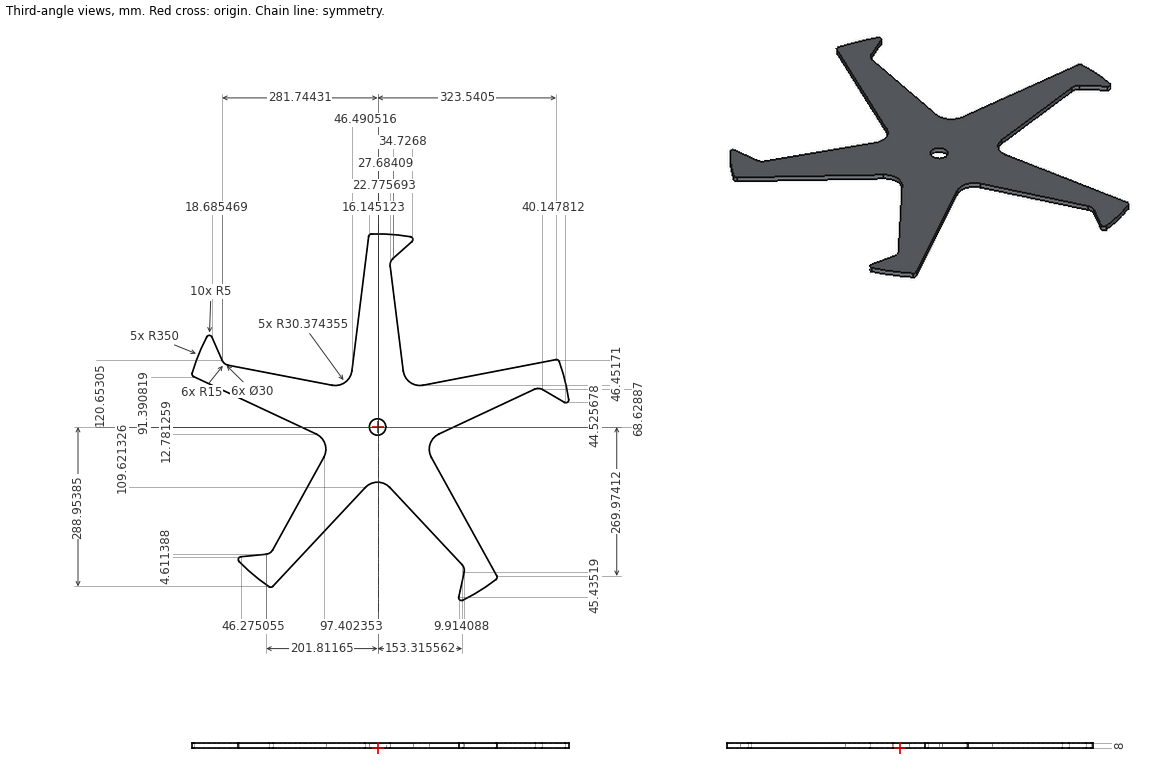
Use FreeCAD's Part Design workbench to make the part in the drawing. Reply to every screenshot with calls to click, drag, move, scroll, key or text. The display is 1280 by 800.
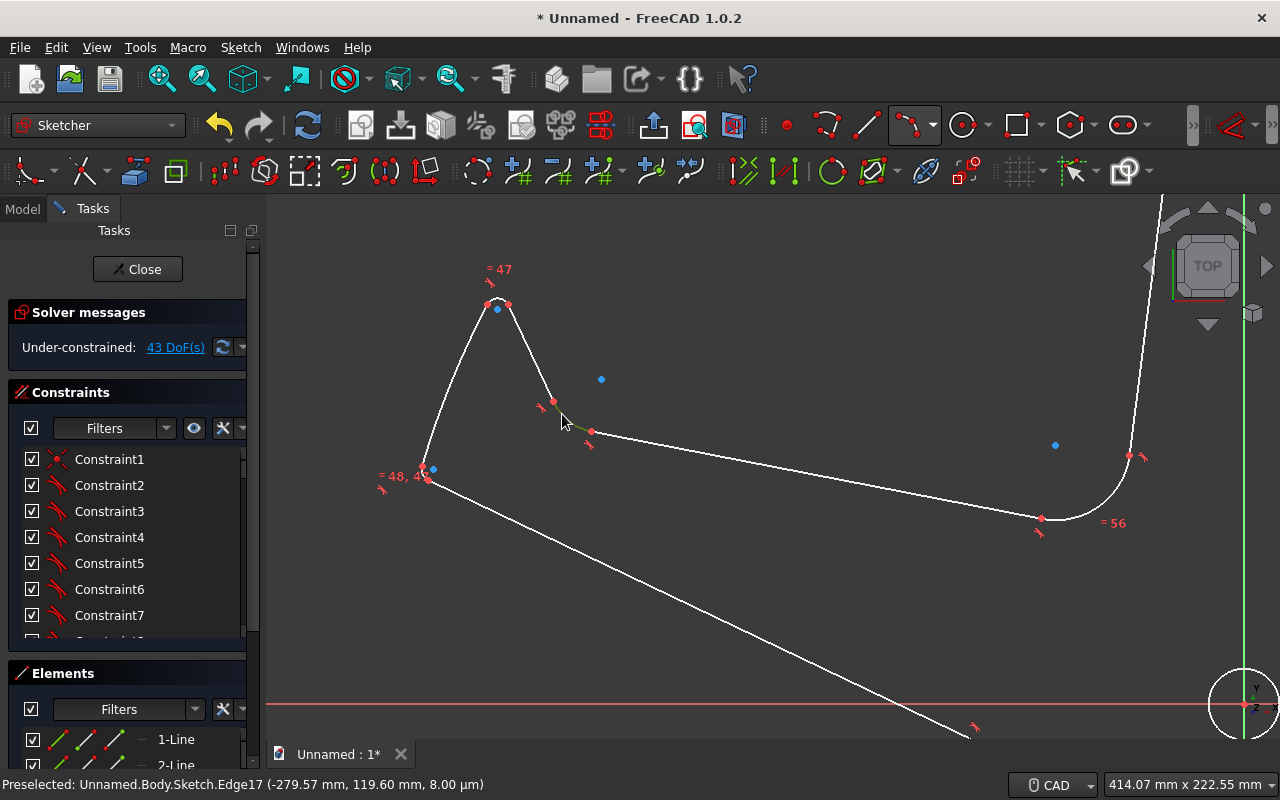
scroll(565, 417, down, 8)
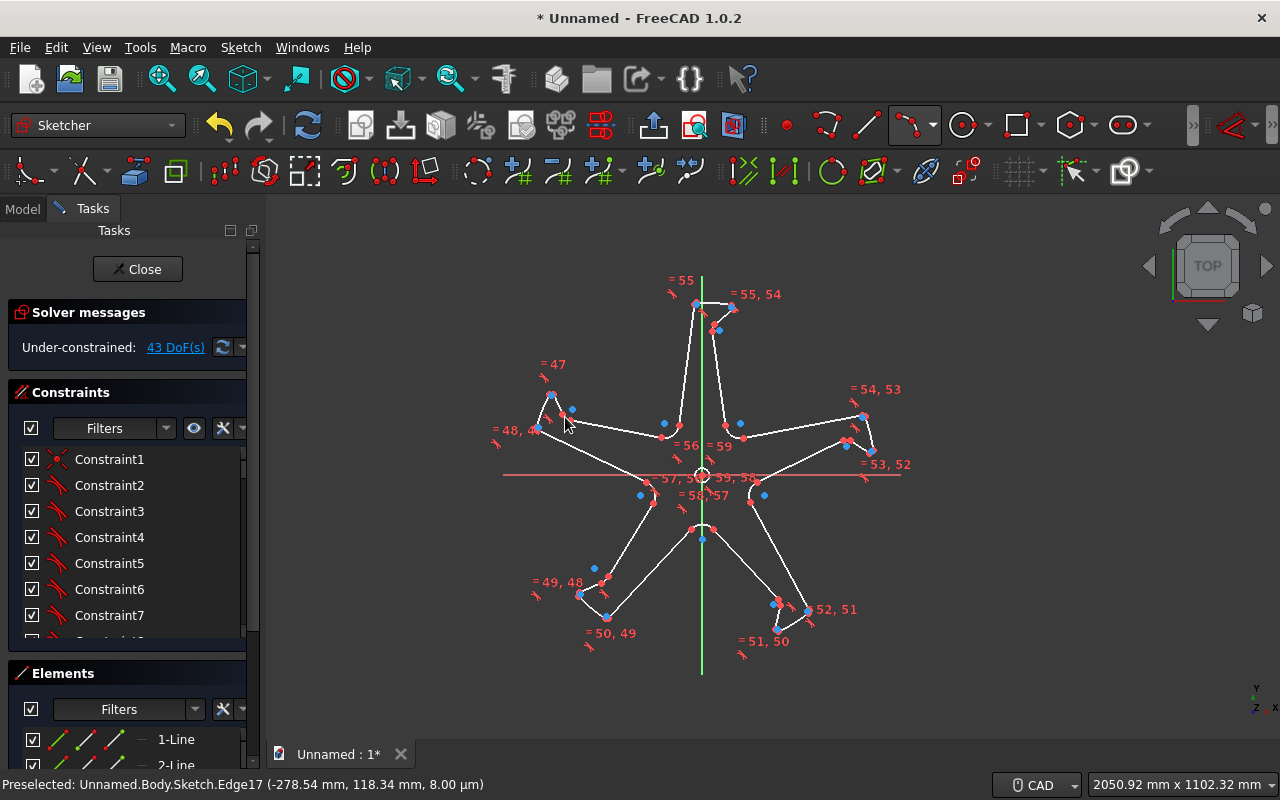
scroll(604, 582, up, 8)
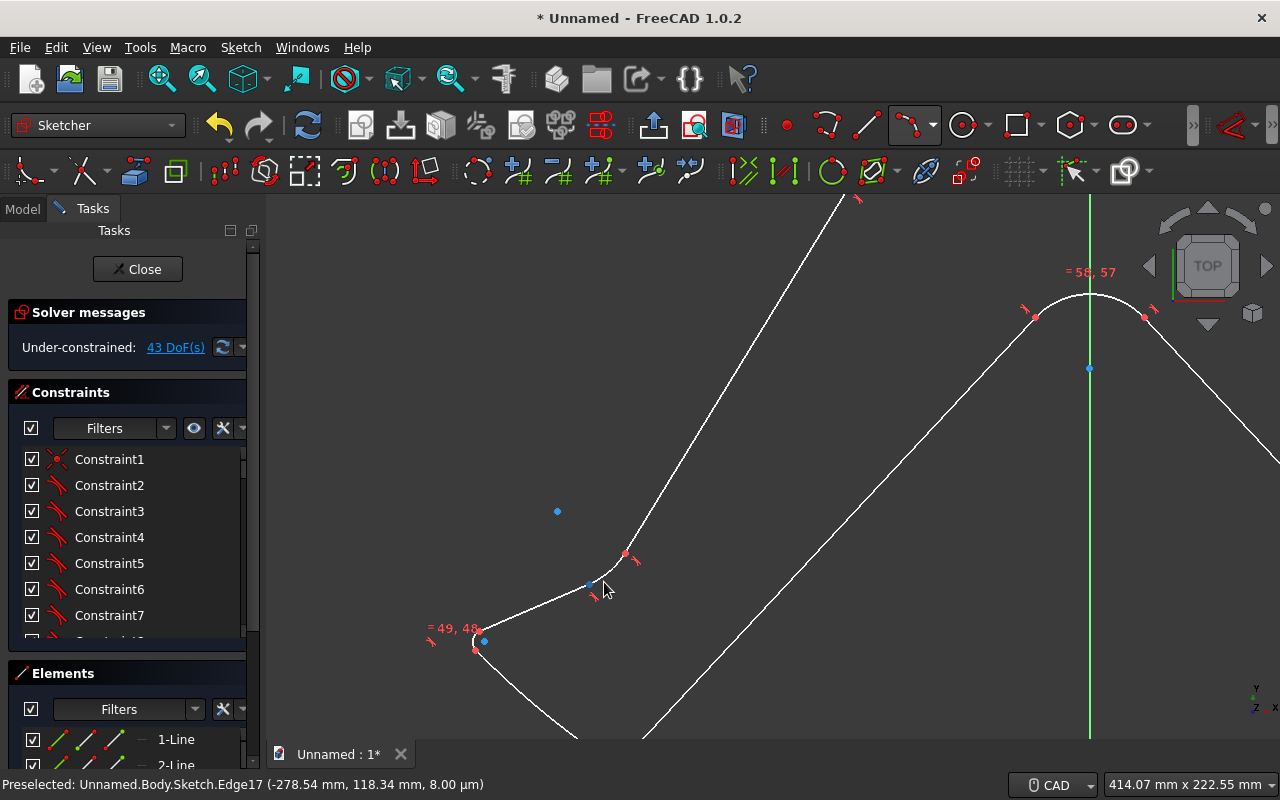
click(602, 577)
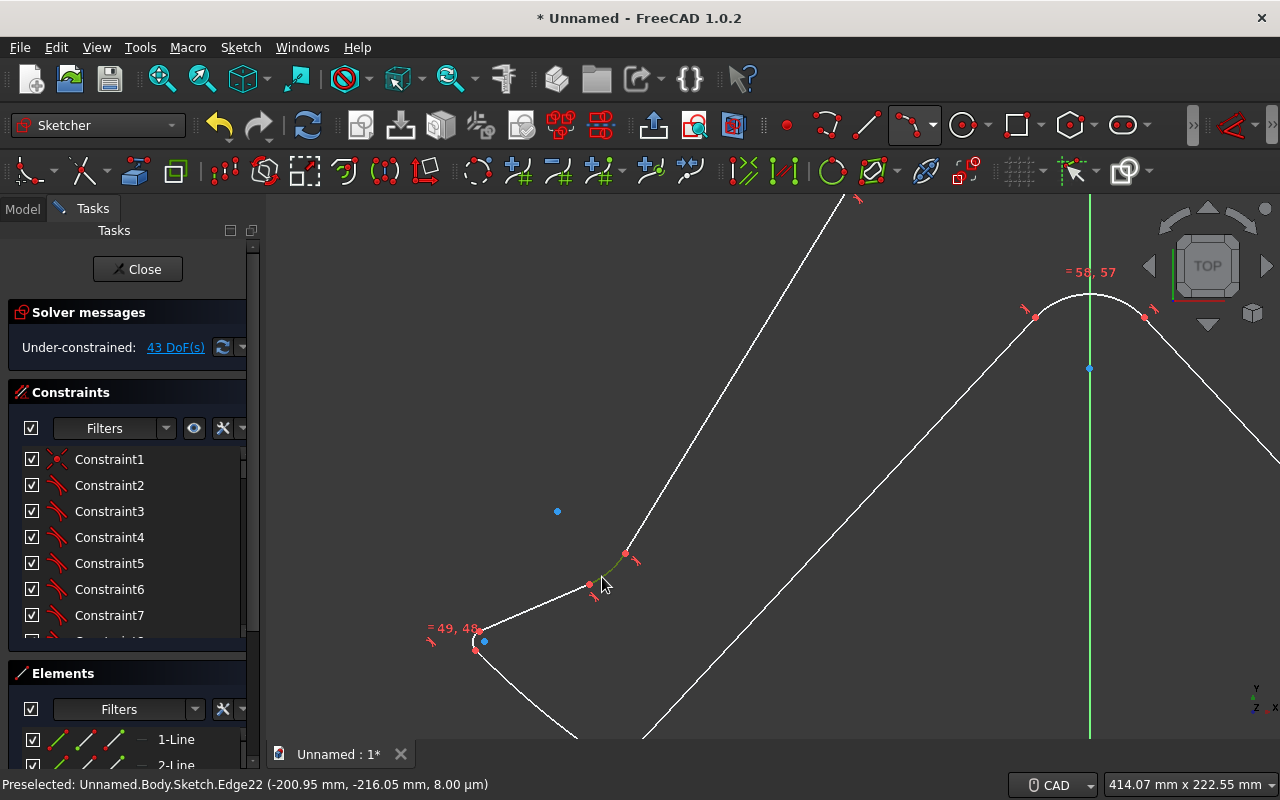
scroll(604, 583, down, 8)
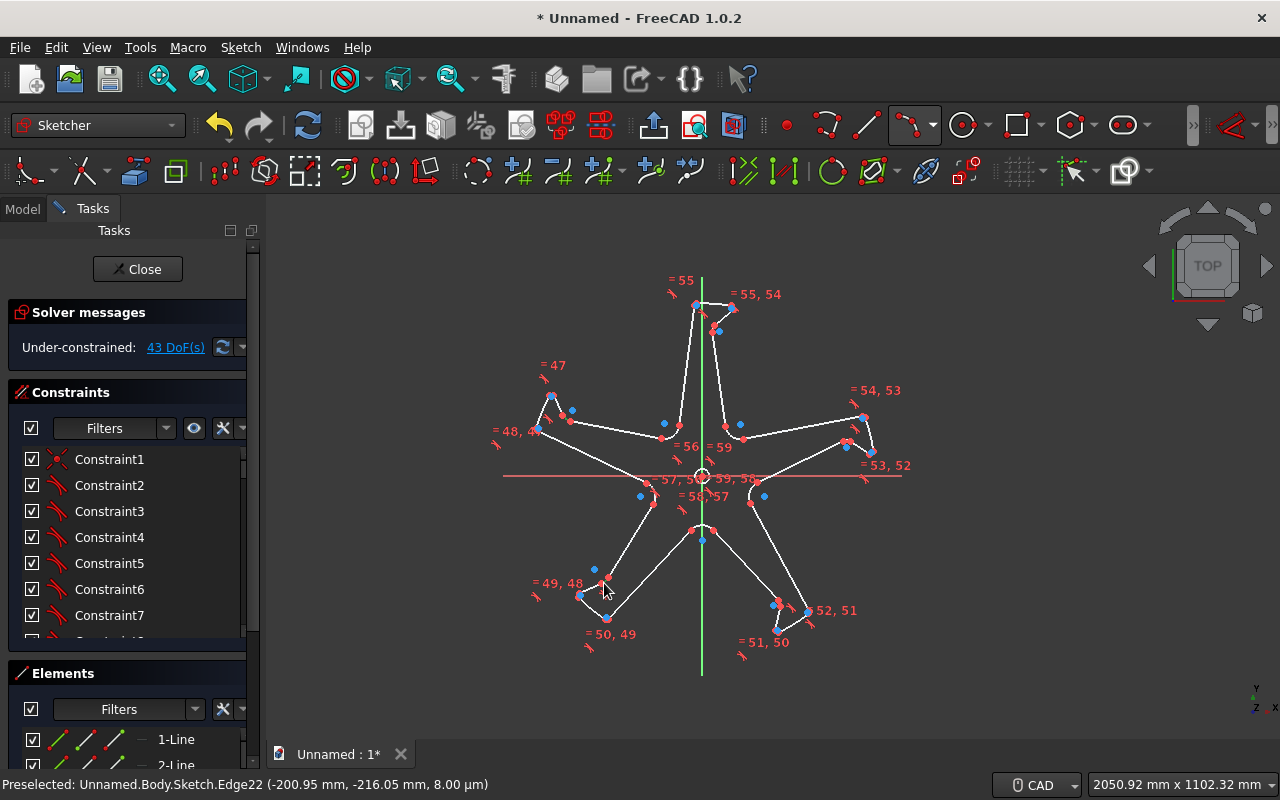
scroll(781, 605, up, 10)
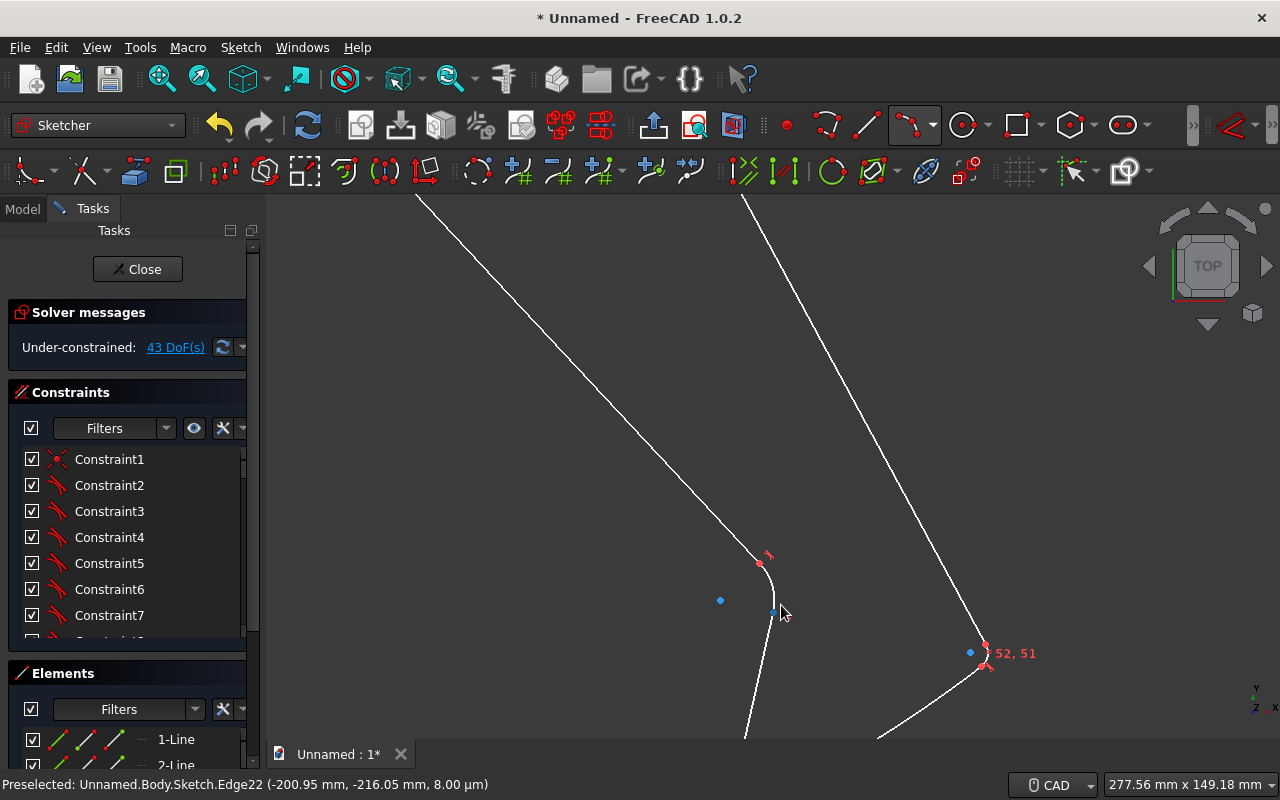
click(774, 597)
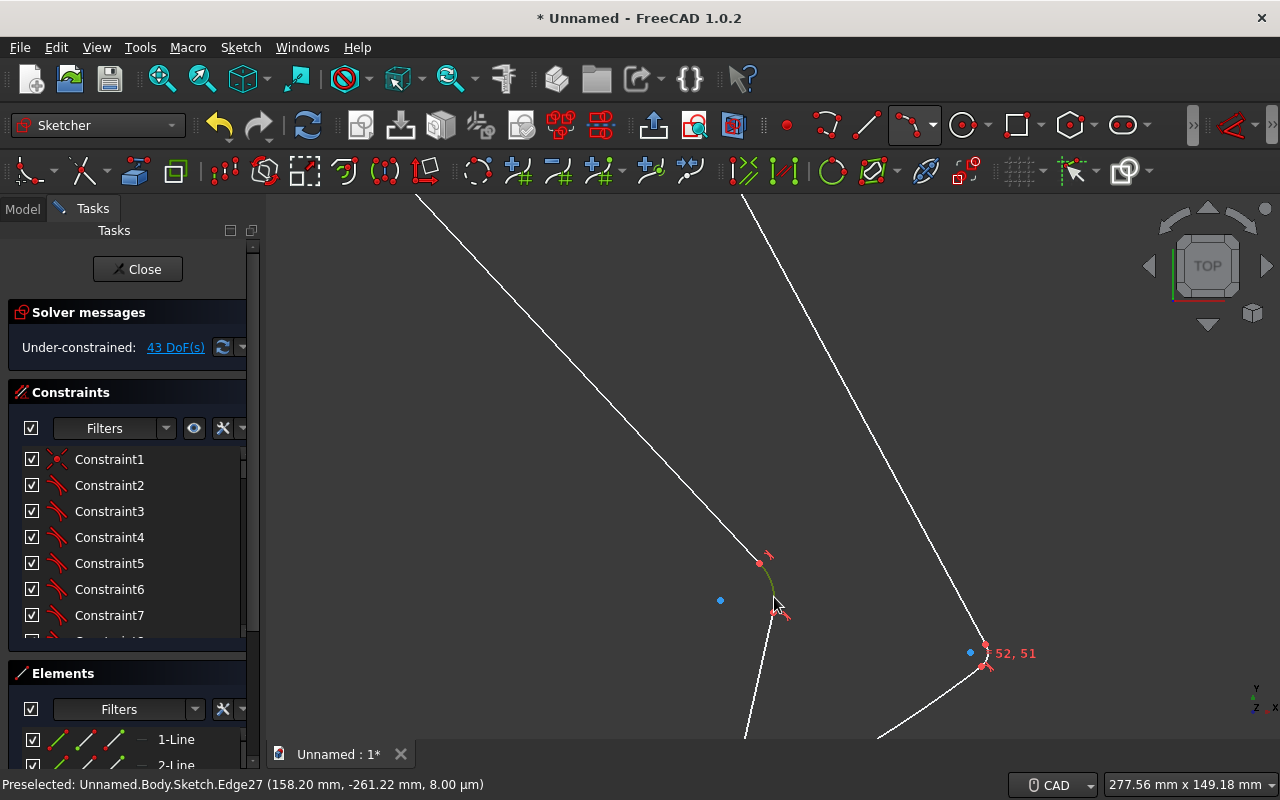
scroll(781, 605, down, 10)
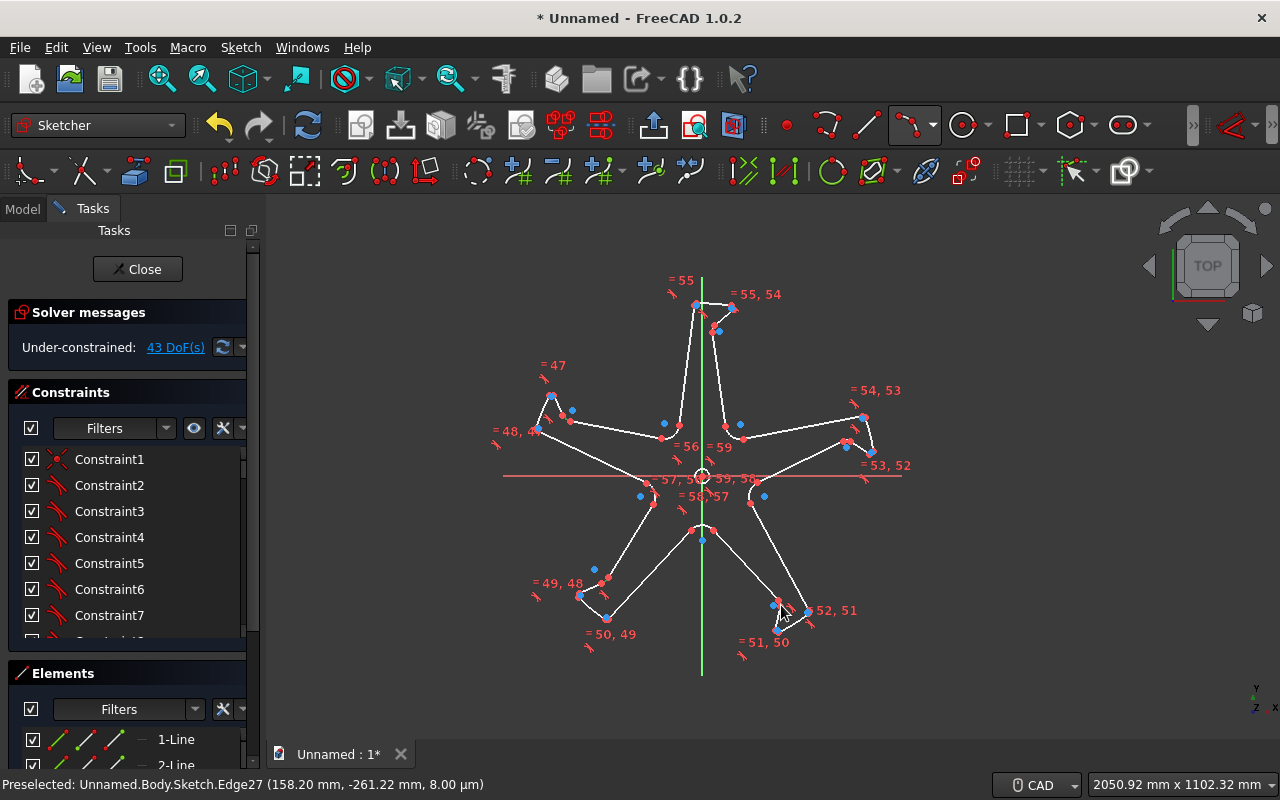
scroll(848, 441, up, 10)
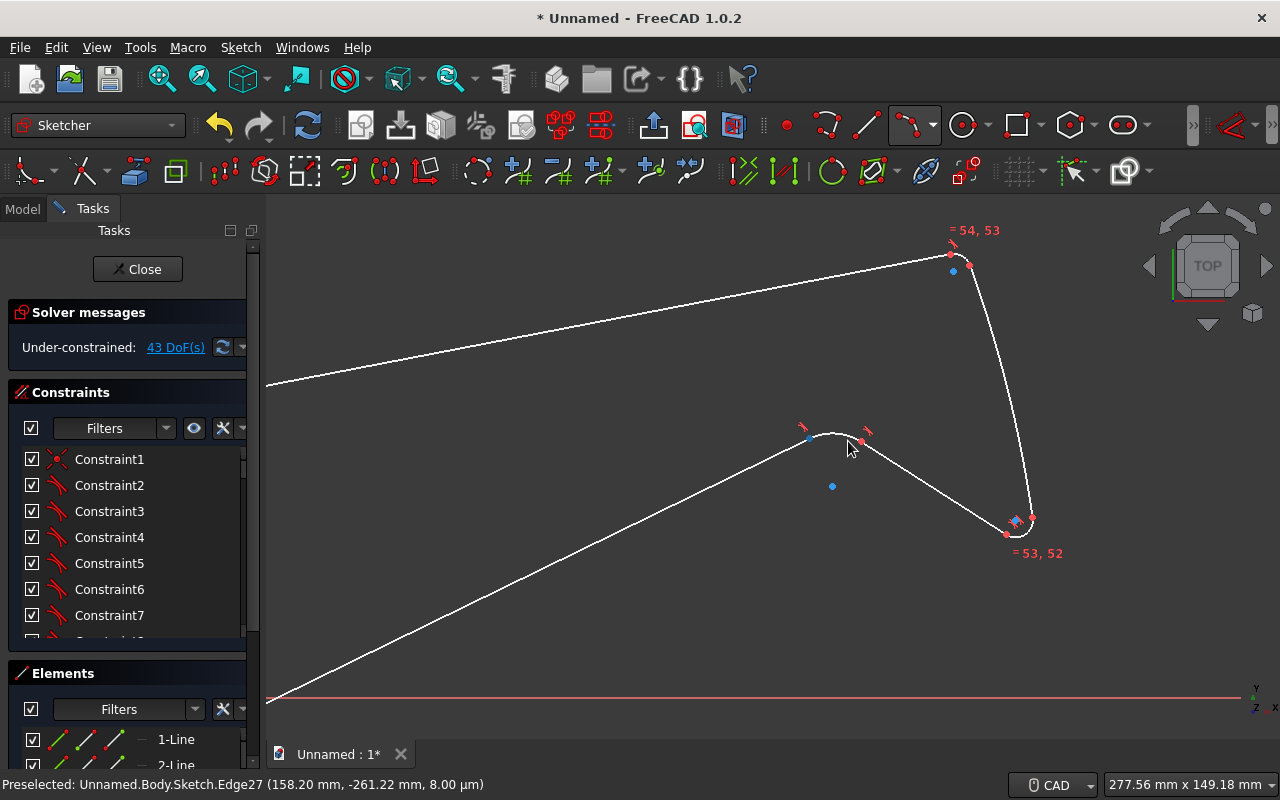
click(846, 435)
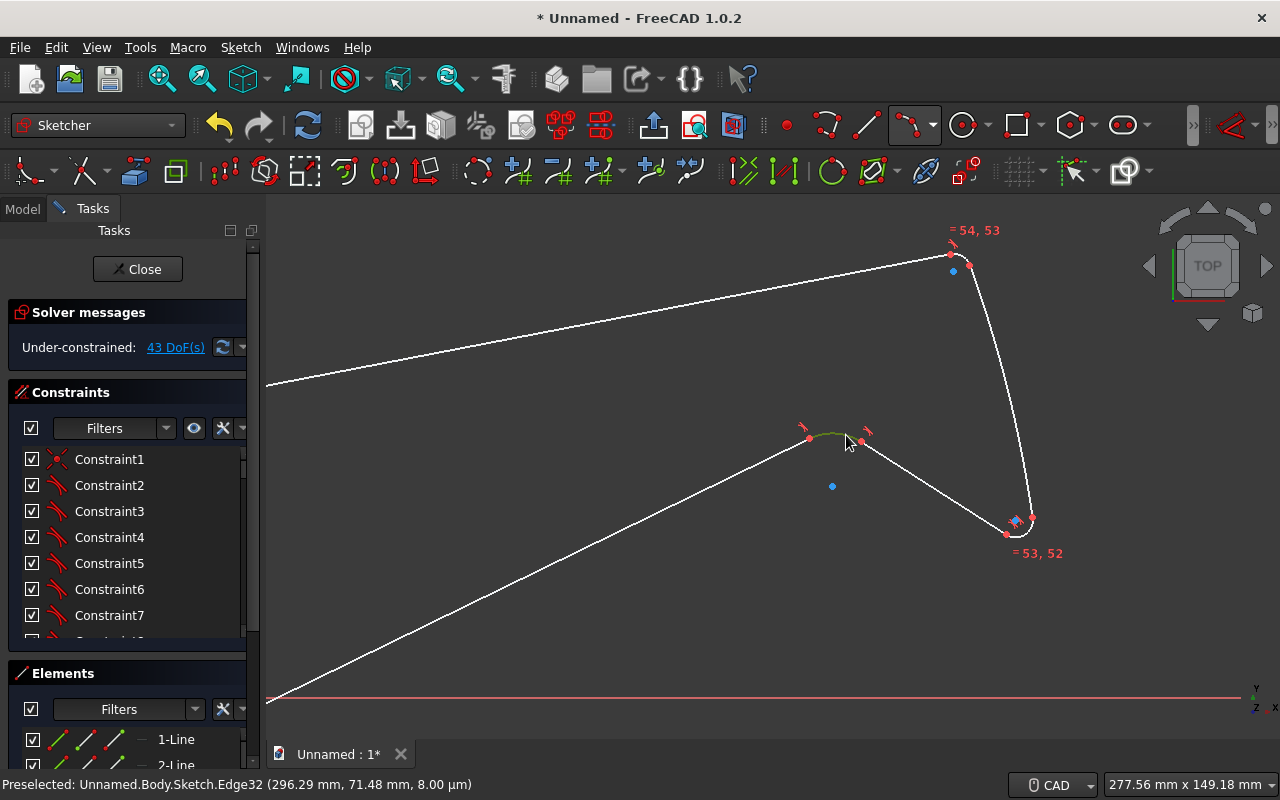
scroll(848, 441, down, 10)